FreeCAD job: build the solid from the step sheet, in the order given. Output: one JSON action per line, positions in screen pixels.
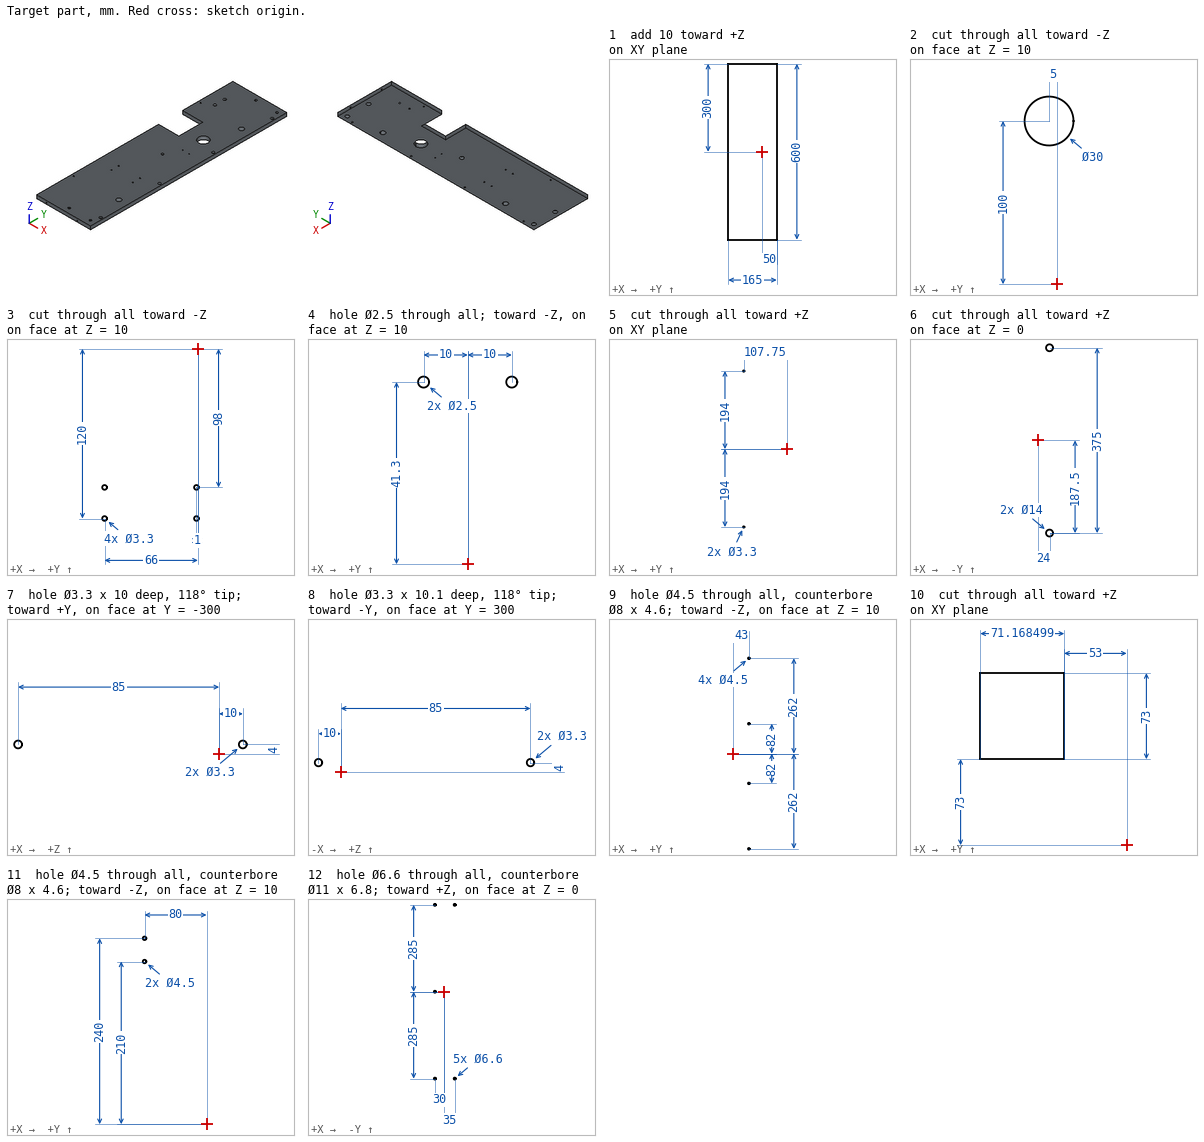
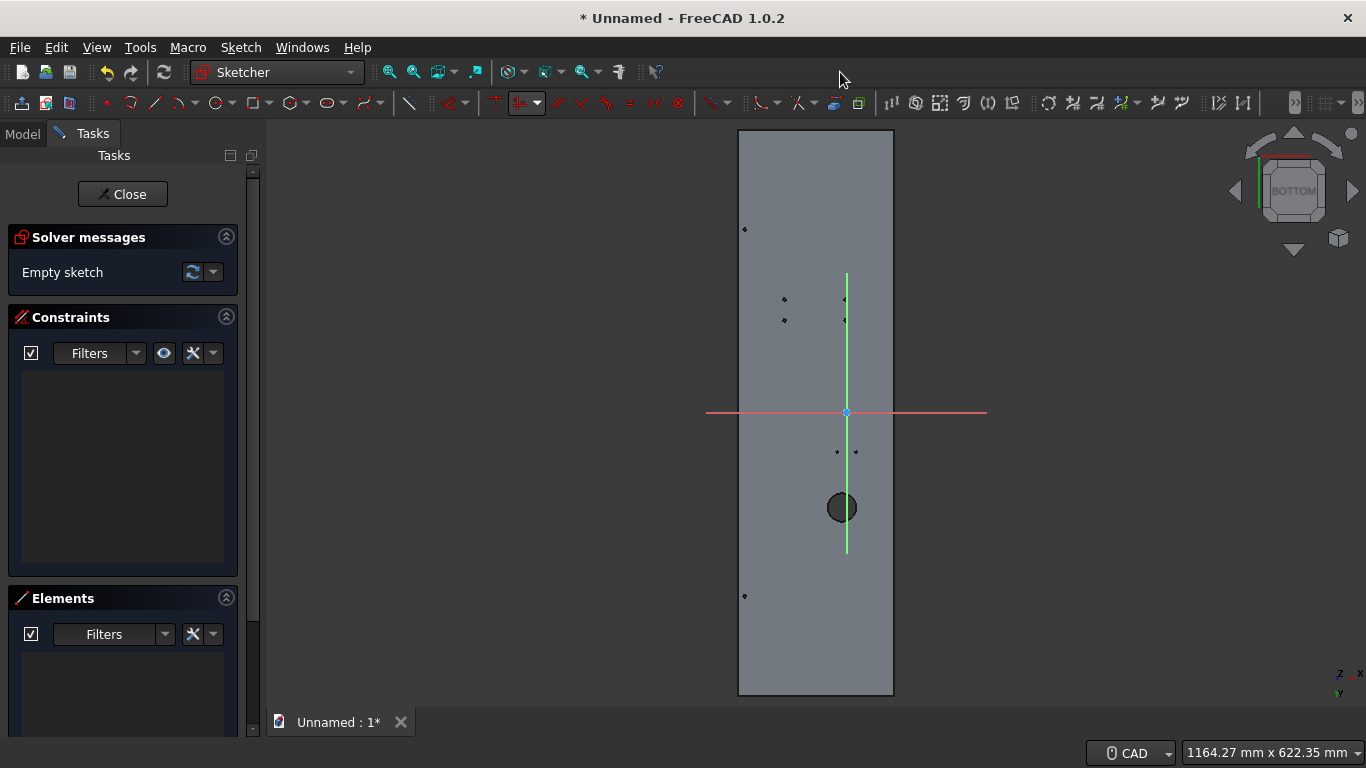
{"action": "left_click", "coordinate": [216, 104]}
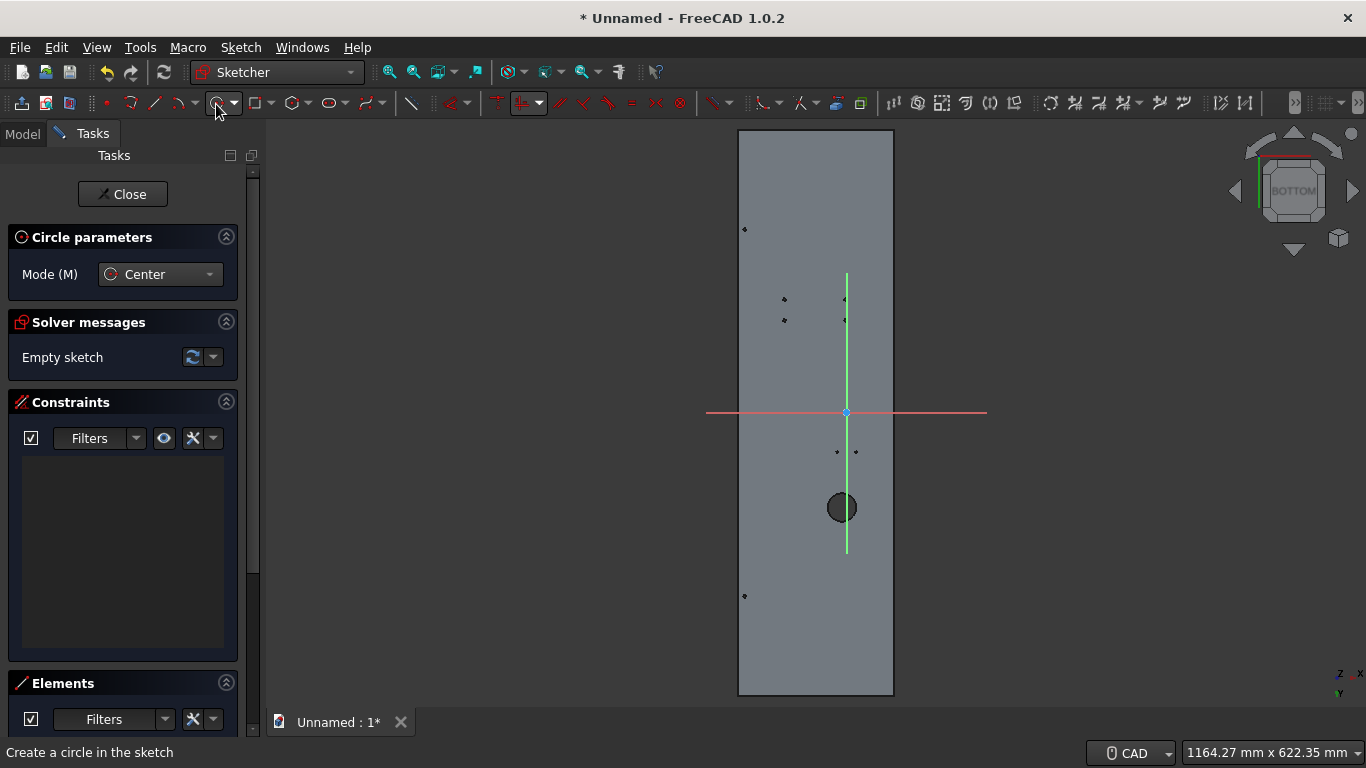
{"action": "scroll", "coordinate": [869, 590], "scroll_direction": "up", "scroll_amount": 7}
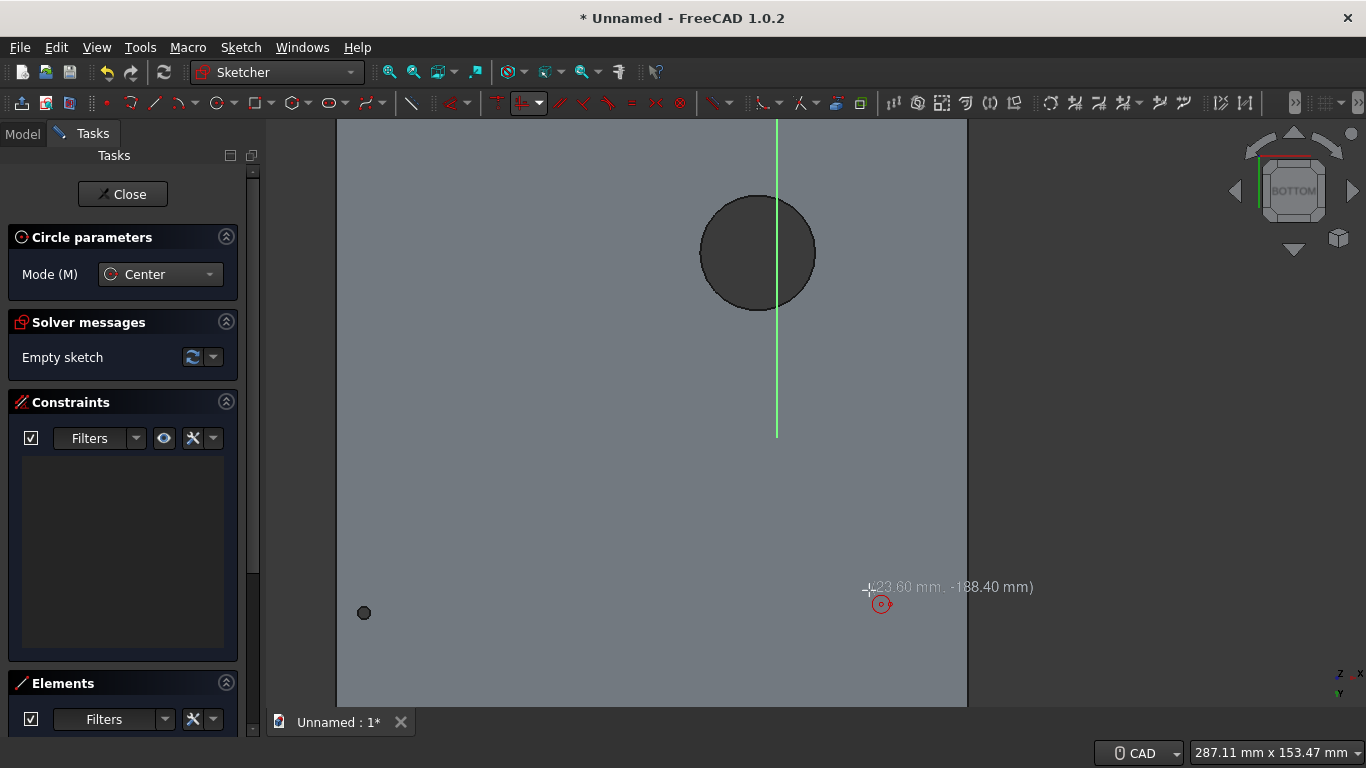
{"action": "scroll", "coordinate": [718, 591], "scroll_direction": "down", "scroll_amount": 7}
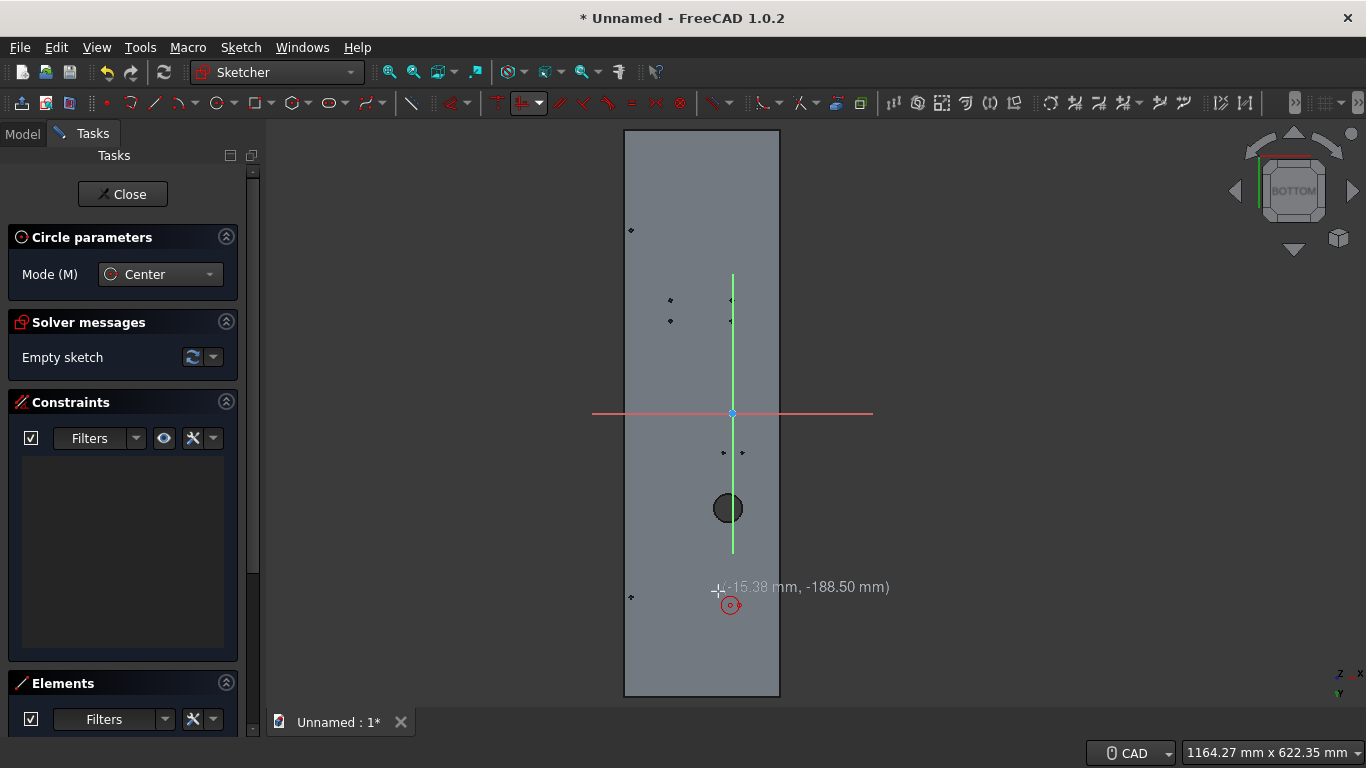
{"action": "left_click", "coordinate": [756, 591]}
{"action": "mouse_move", "coordinate": [760, 586]}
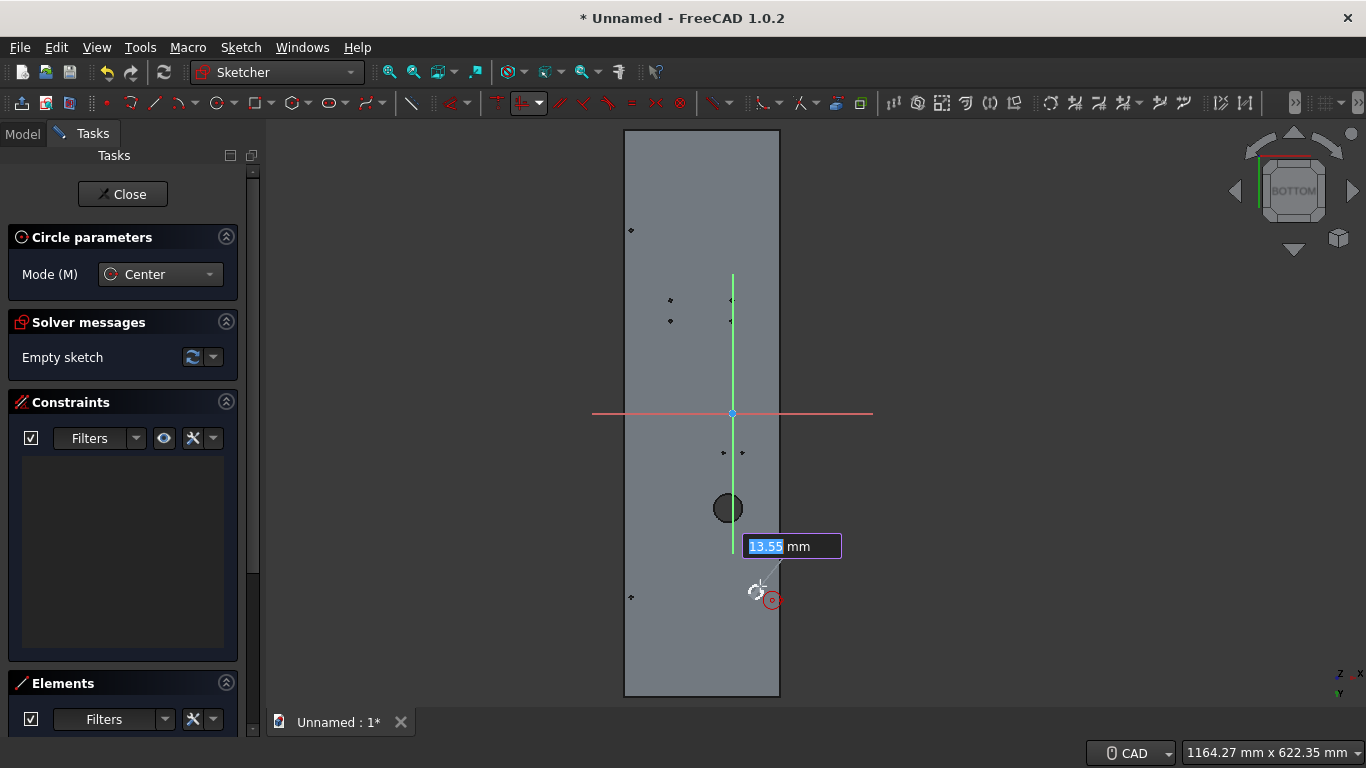
{"action": "type", "text": "14"}
{"action": "key", "text": "Return"}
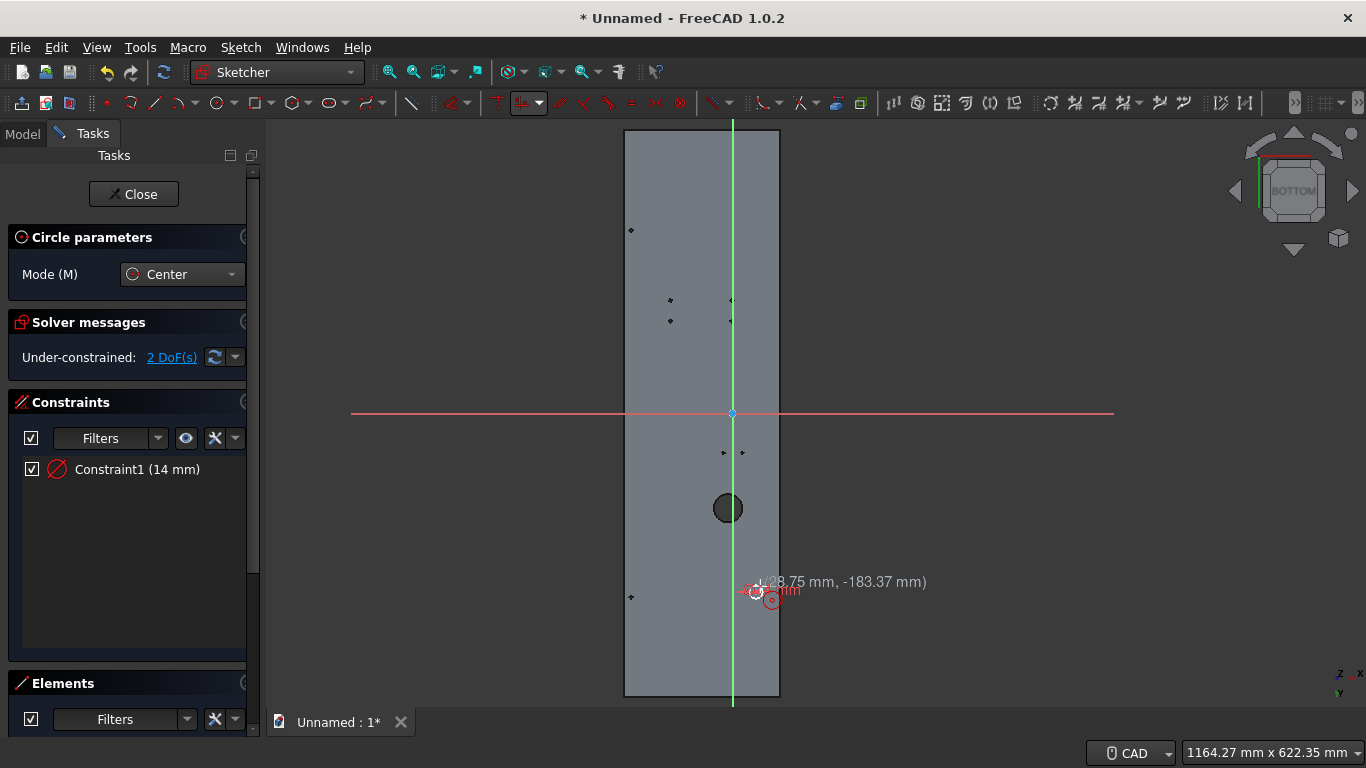
{"action": "scroll", "coordinate": [756, 237], "scroll_direction": "up", "scroll_amount": 7}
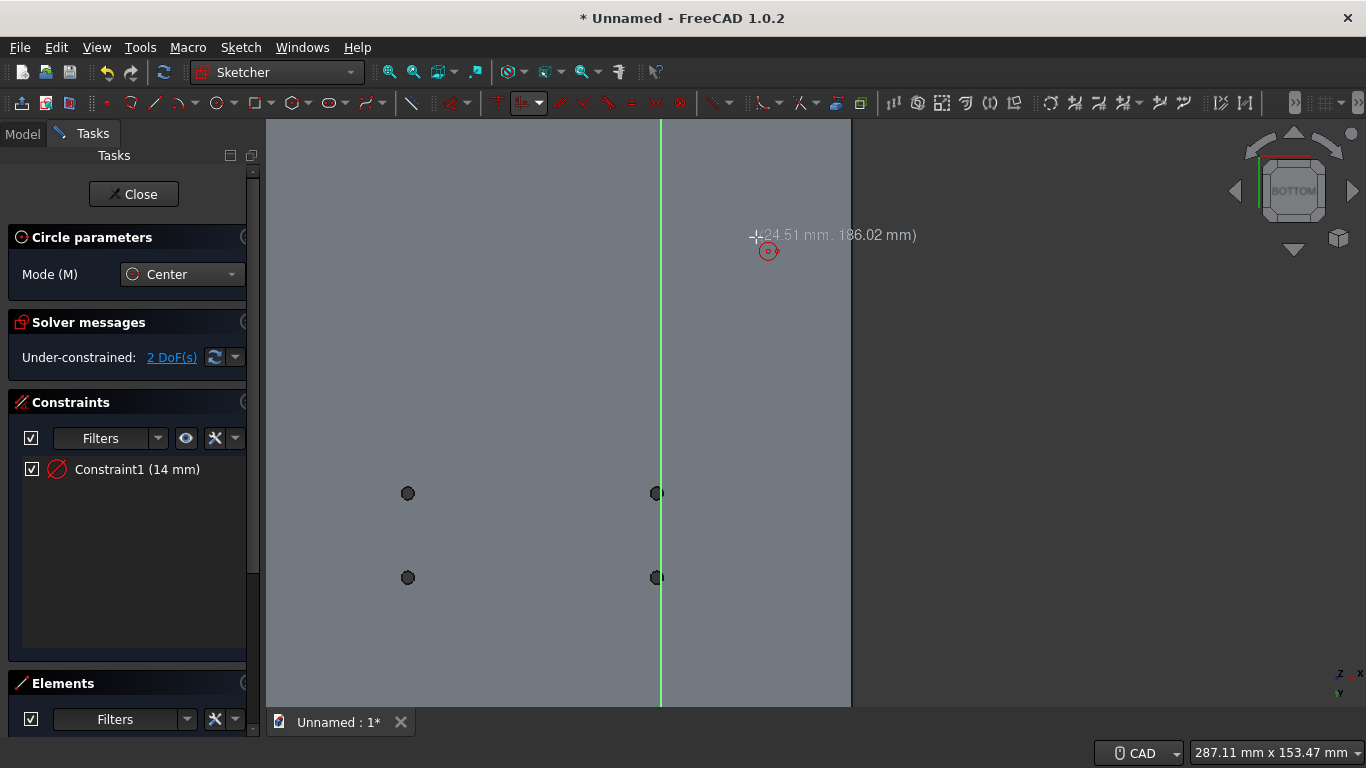
{"action": "scroll", "coordinate": [756, 236], "scroll_direction": "down", "scroll_amount": 7}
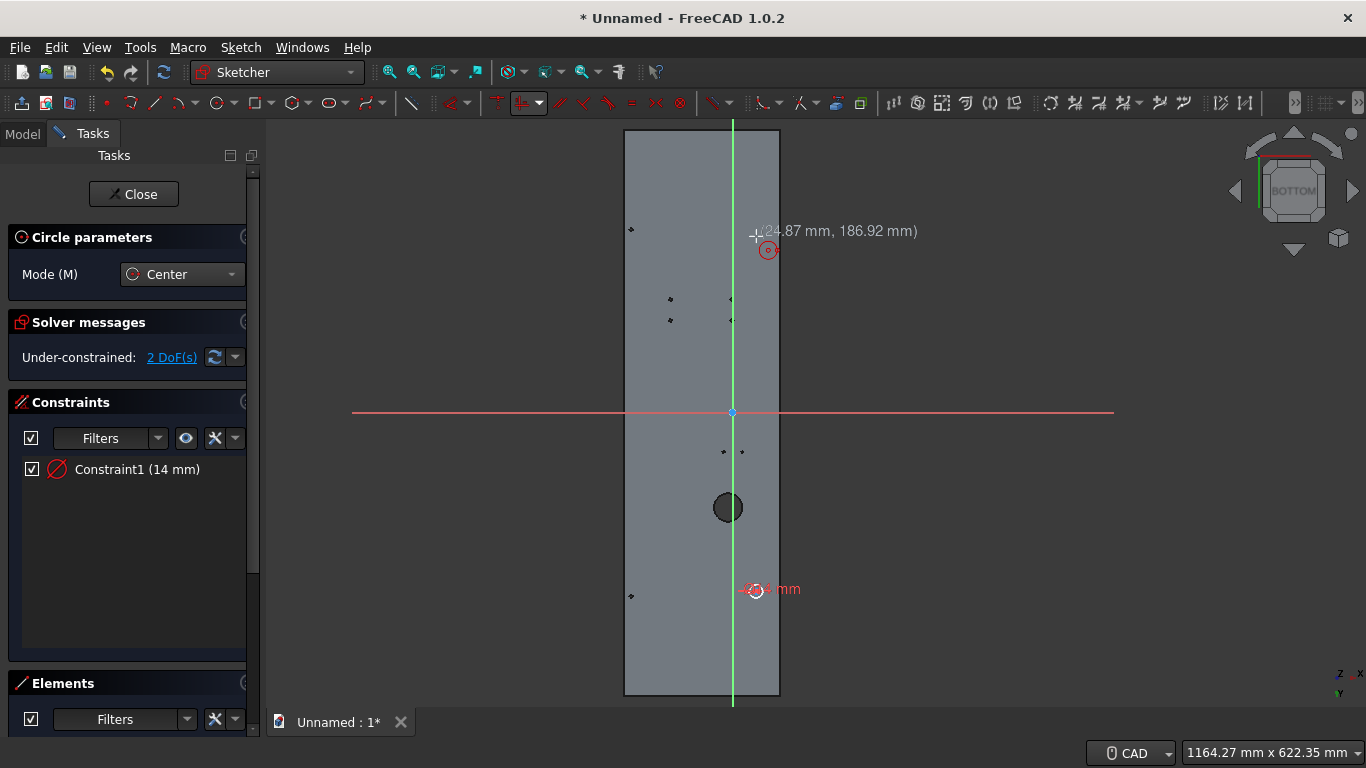
{"action": "left_click", "coordinate": [756, 236]}
{"action": "mouse_move", "coordinate": [760, 231]}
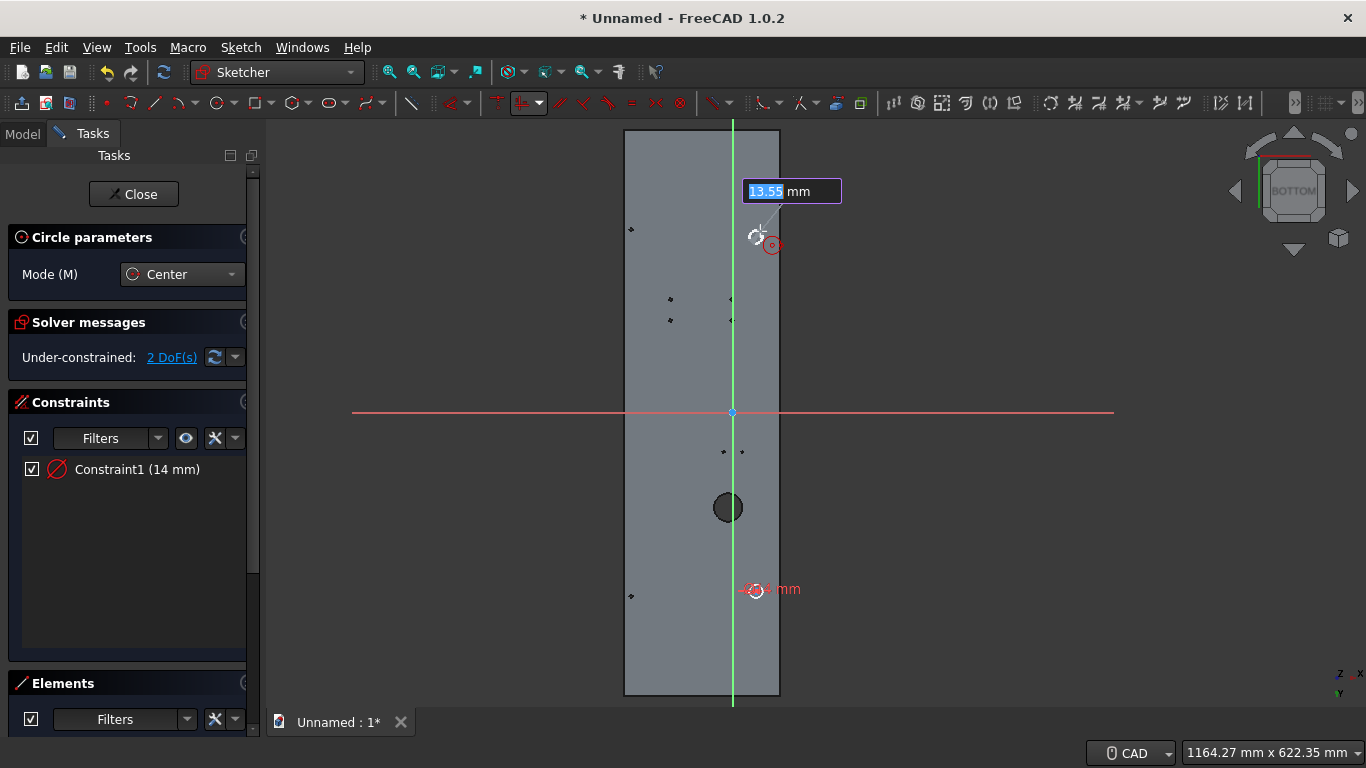
{"action": "type", "text": "14"}
{"action": "key", "text": "Return"}
{"action": "key", "text": "Escape"}